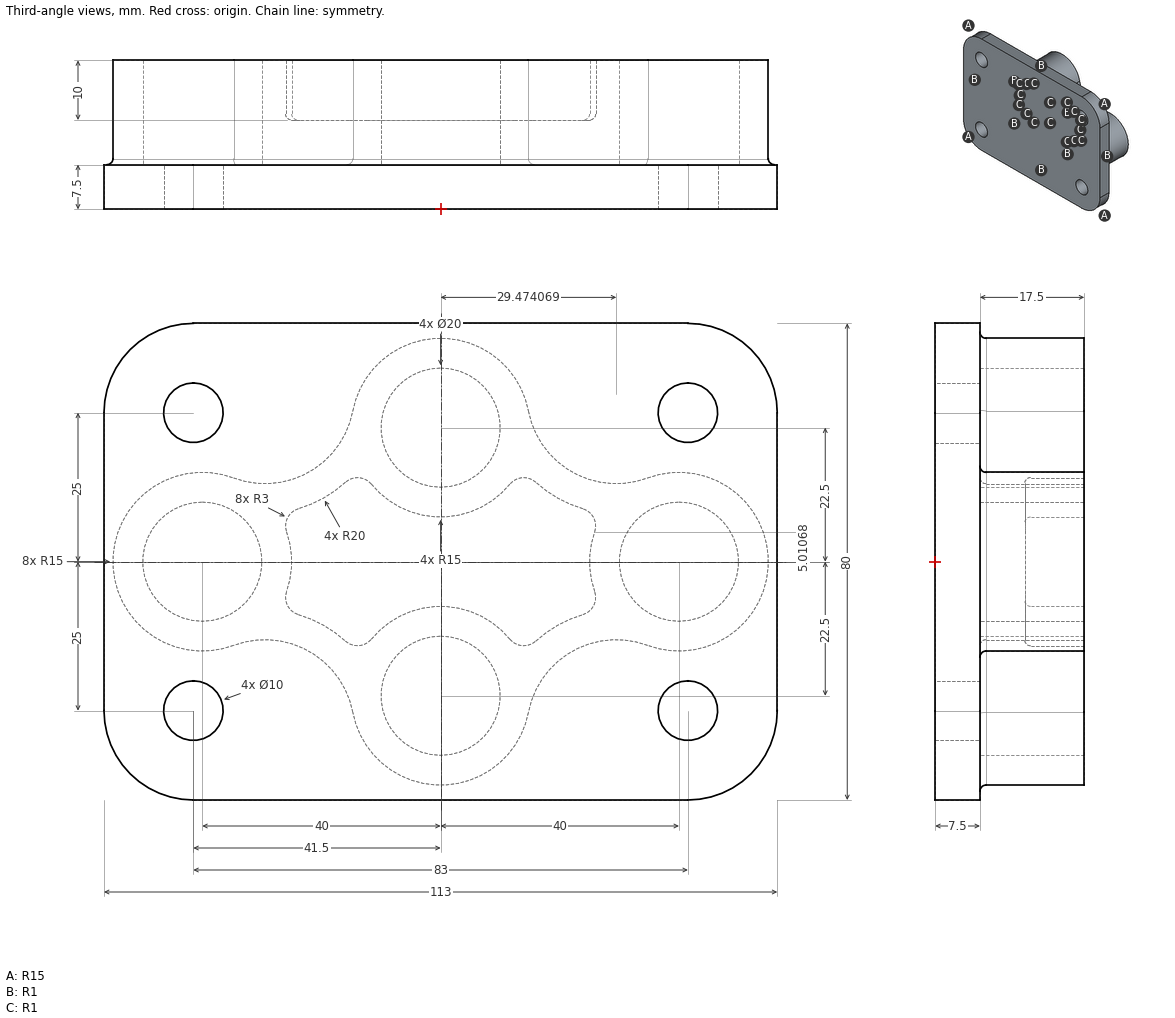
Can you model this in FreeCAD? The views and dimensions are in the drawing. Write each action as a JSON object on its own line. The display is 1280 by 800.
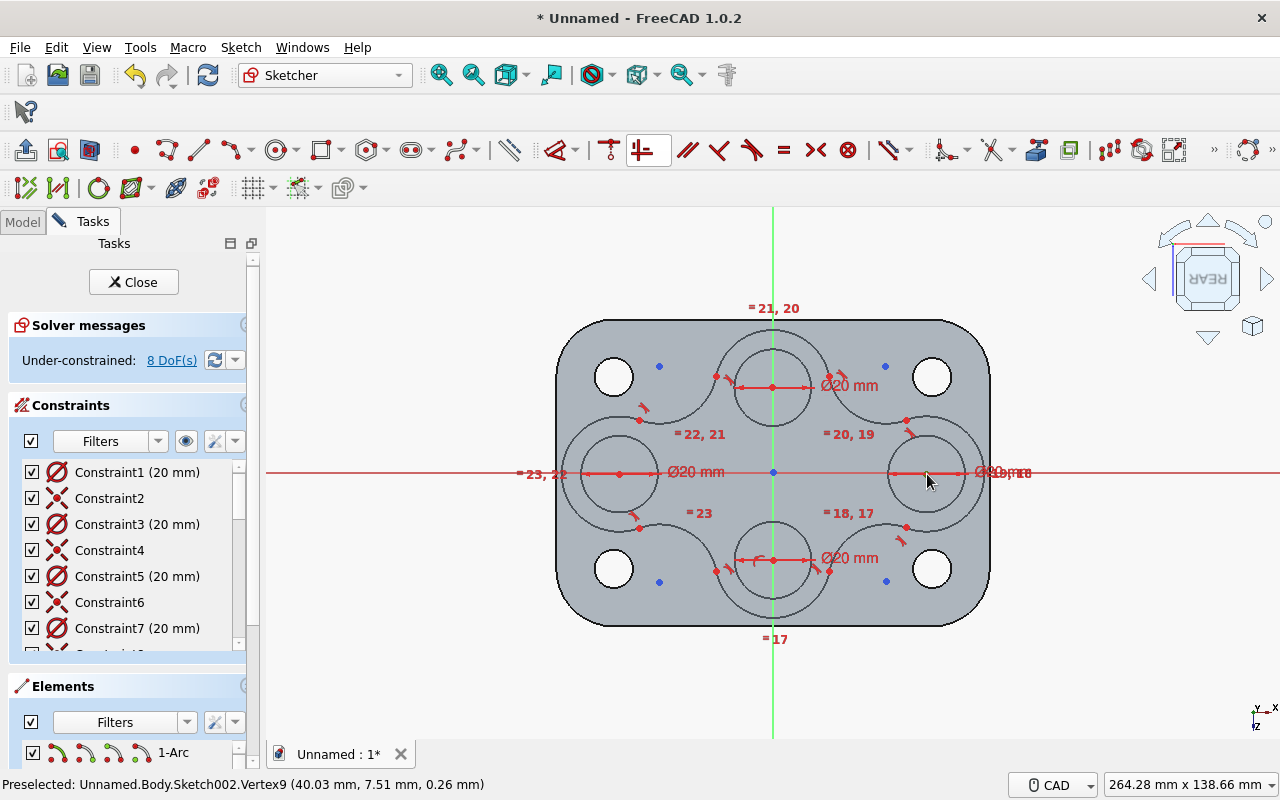
{"action": "left_click", "coordinate": [353, 473]}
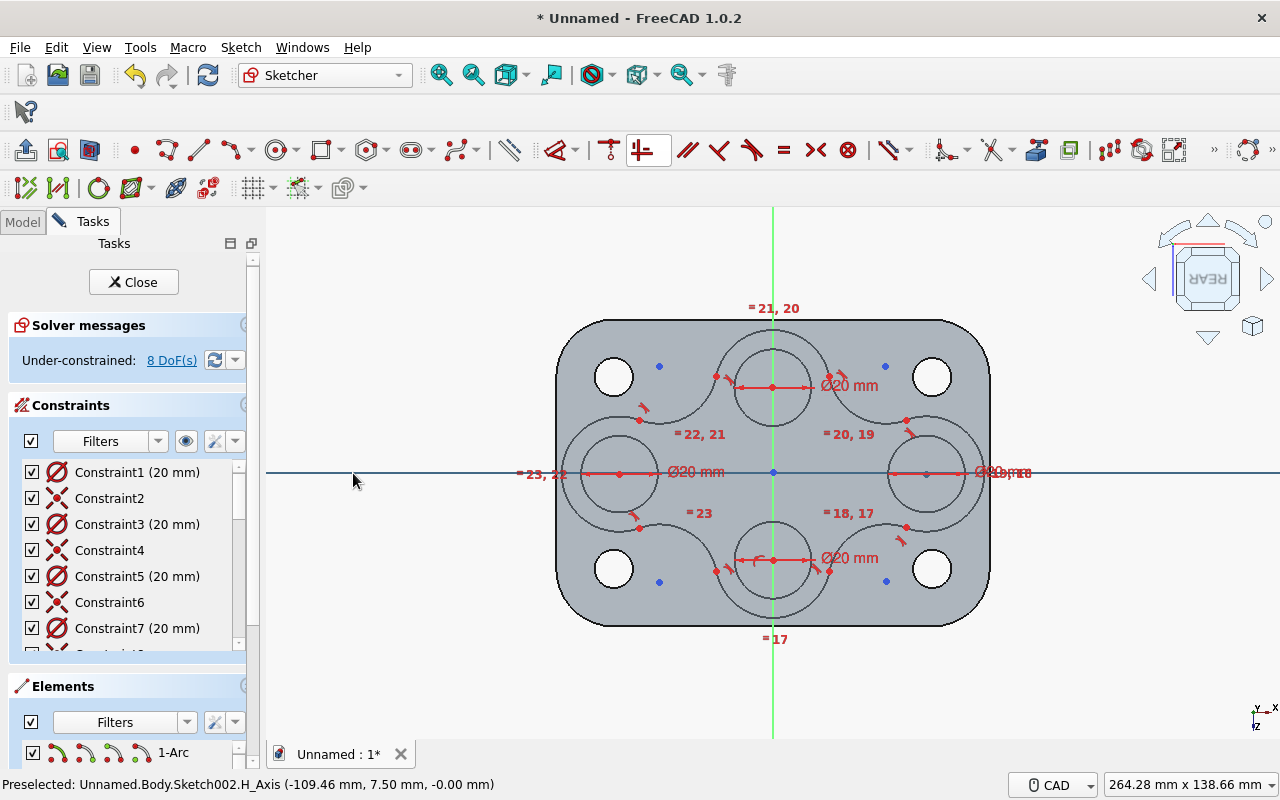
{"action": "left_click", "coordinate": [610, 150]}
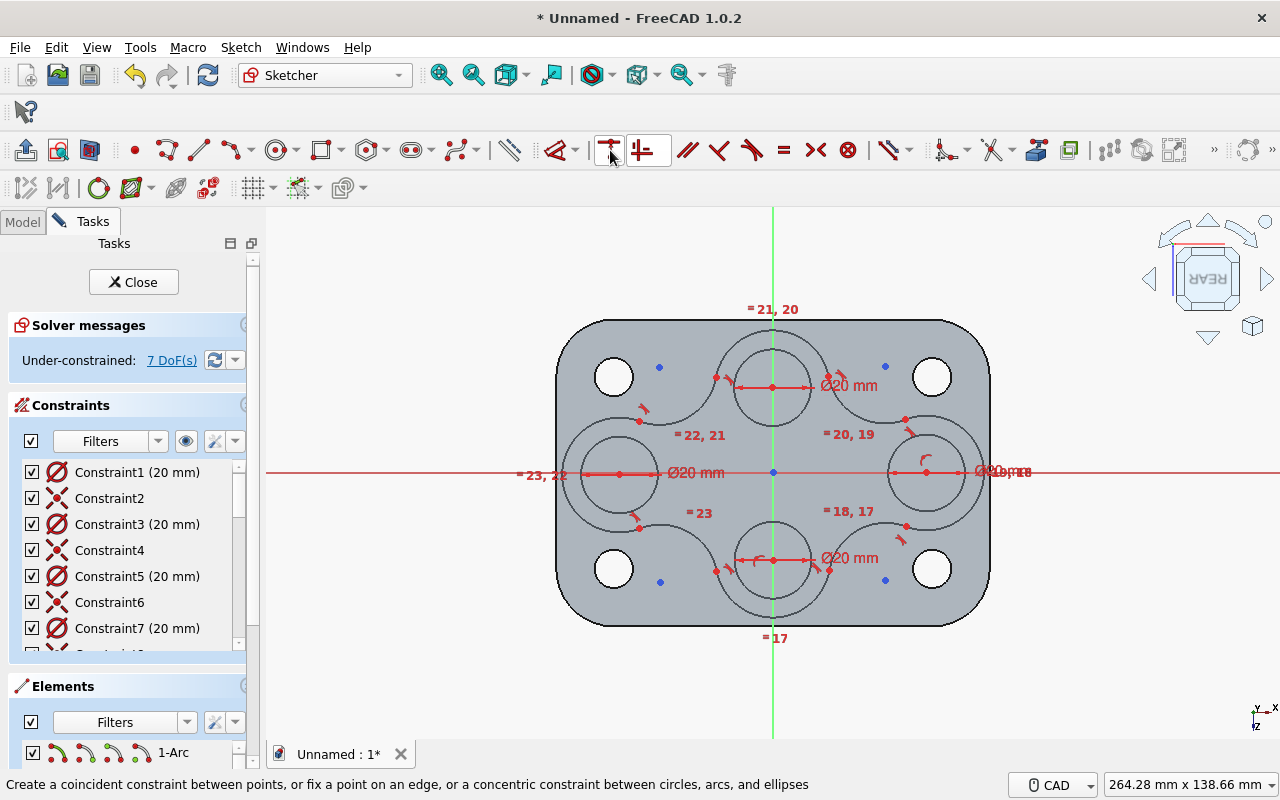
{"action": "left_click", "coordinate": [772, 388]}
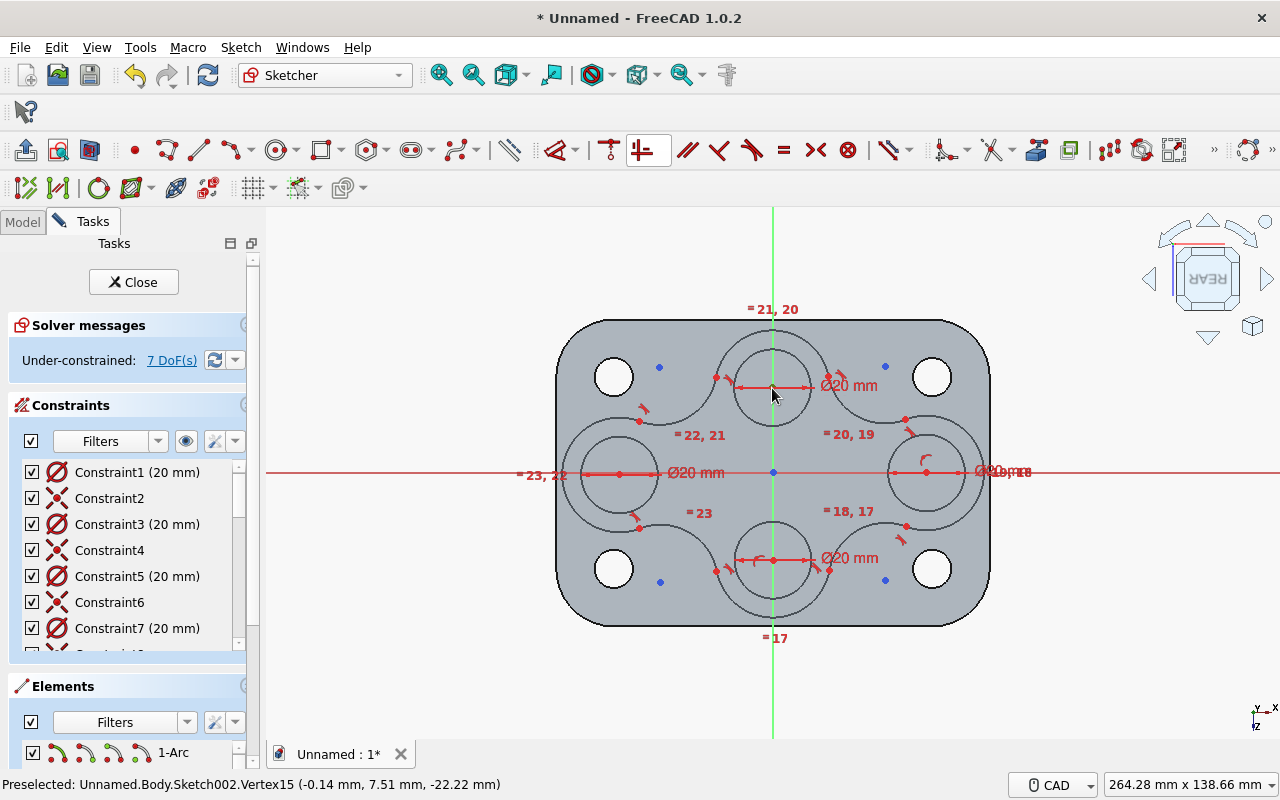
{"action": "left_click", "coordinate": [773, 677]}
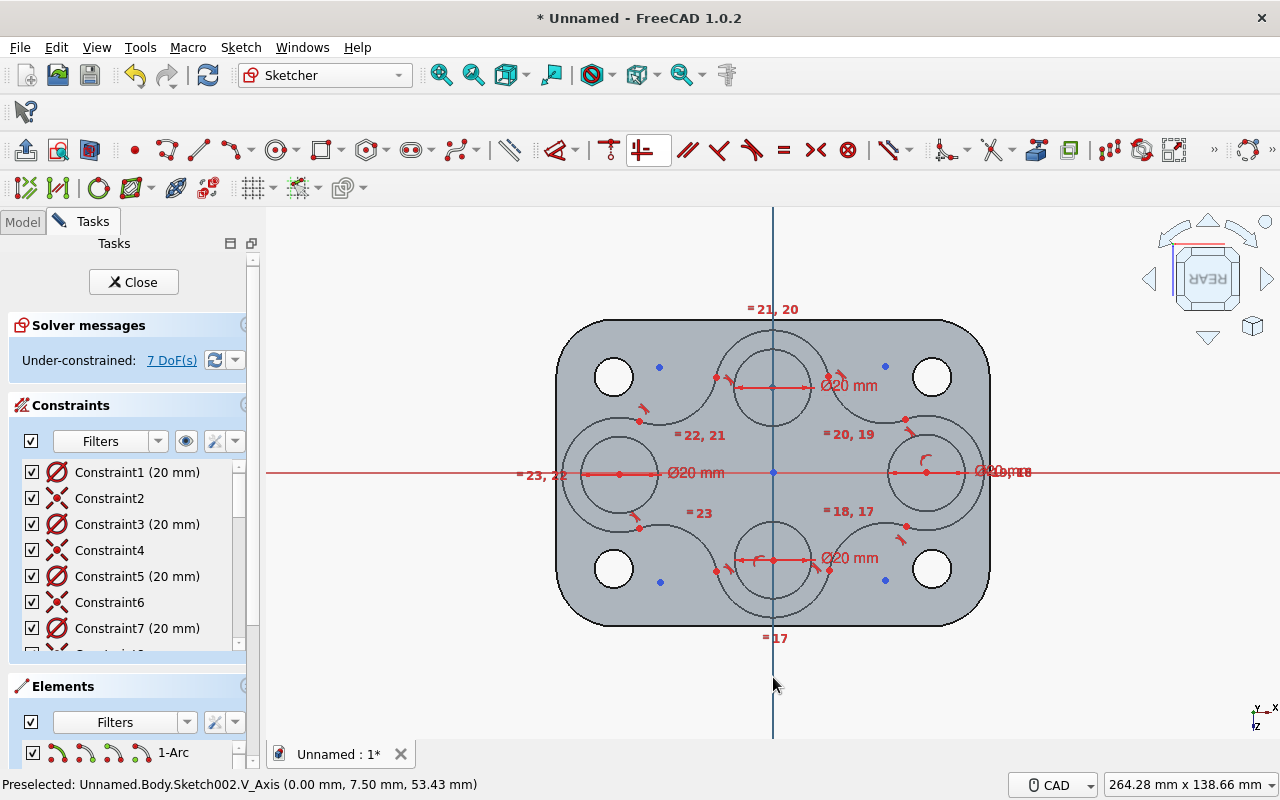
{"action": "left_click", "coordinate": [610, 150]}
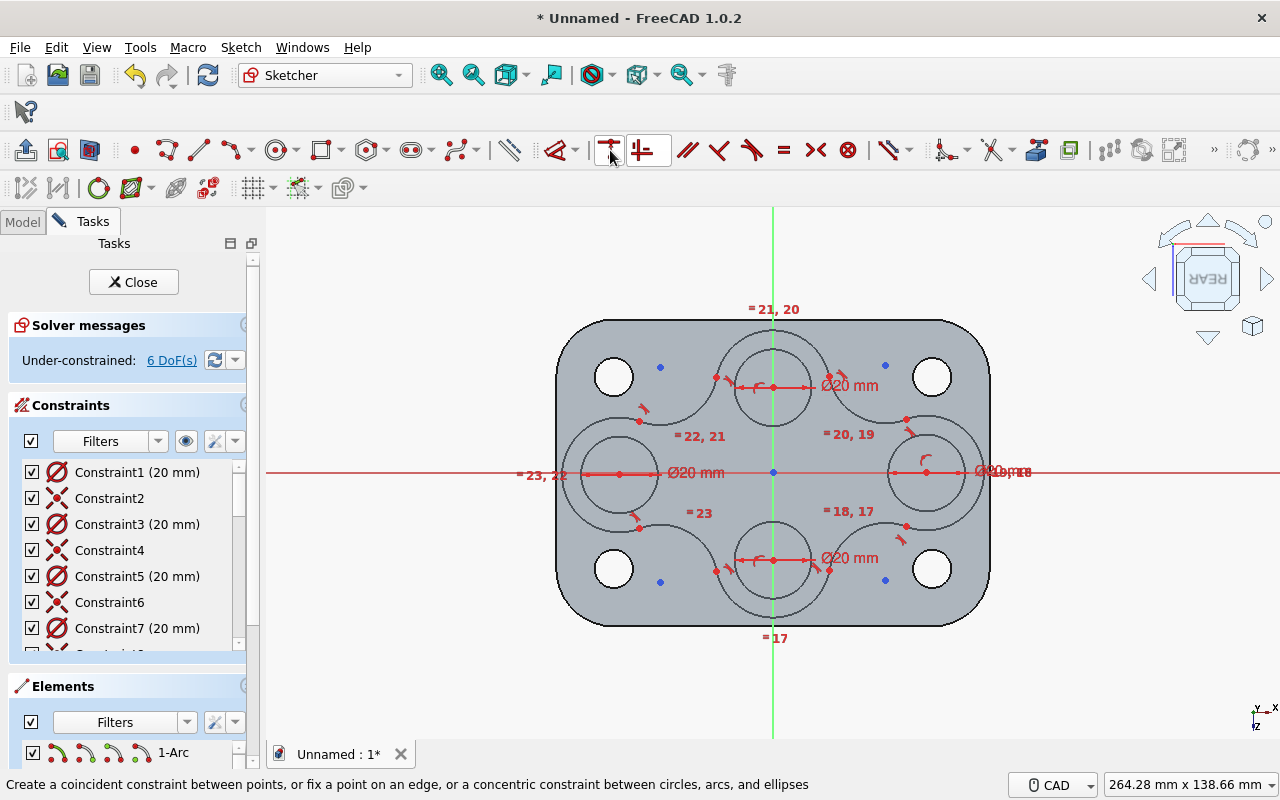
{"action": "left_click", "coordinate": [619, 475]}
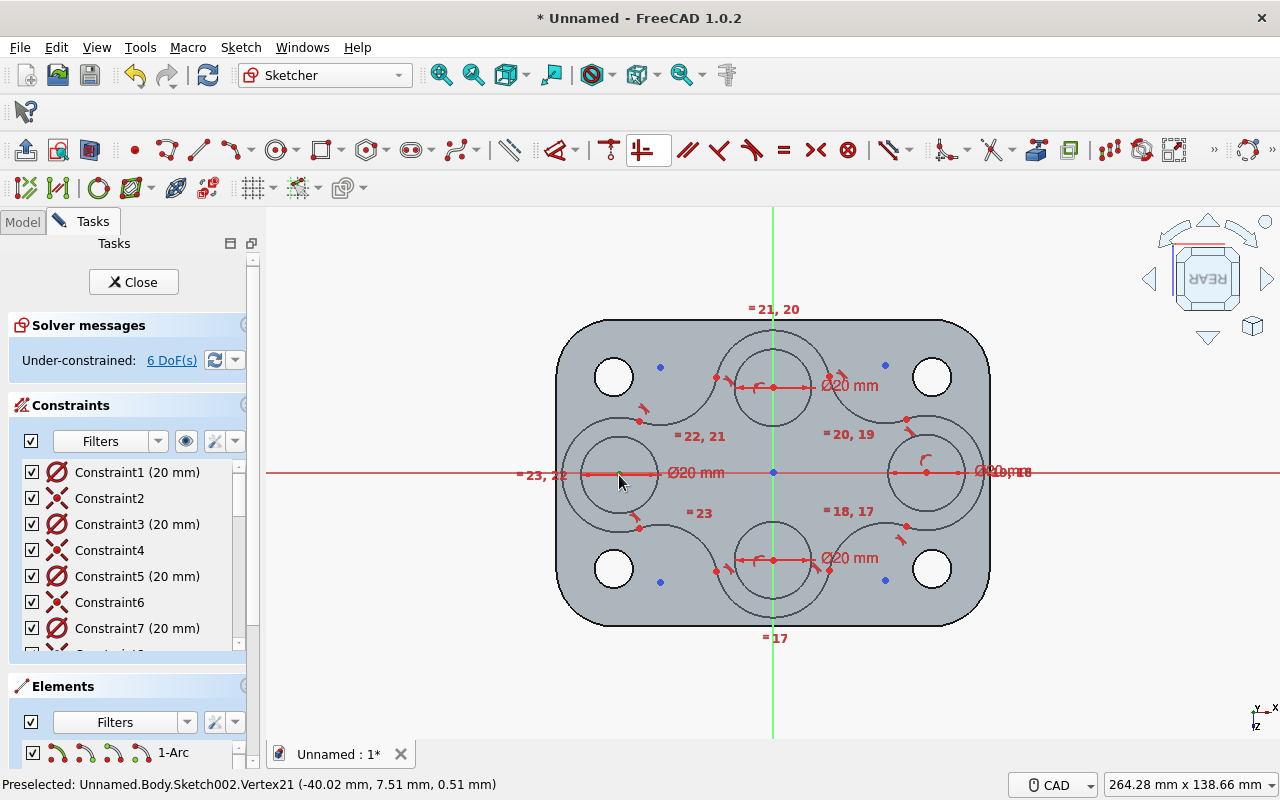
{"action": "left_click", "coordinate": [353, 473]}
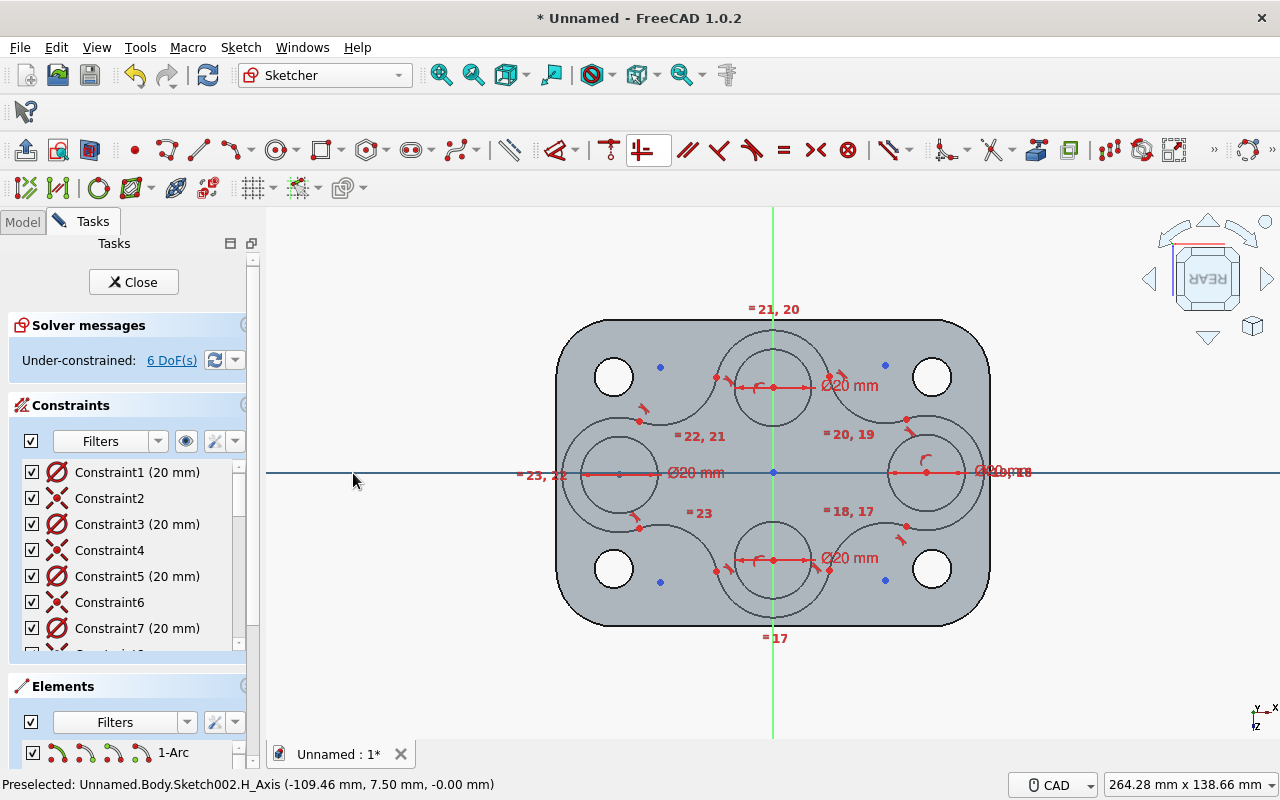
{"action": "key", "text": "c"}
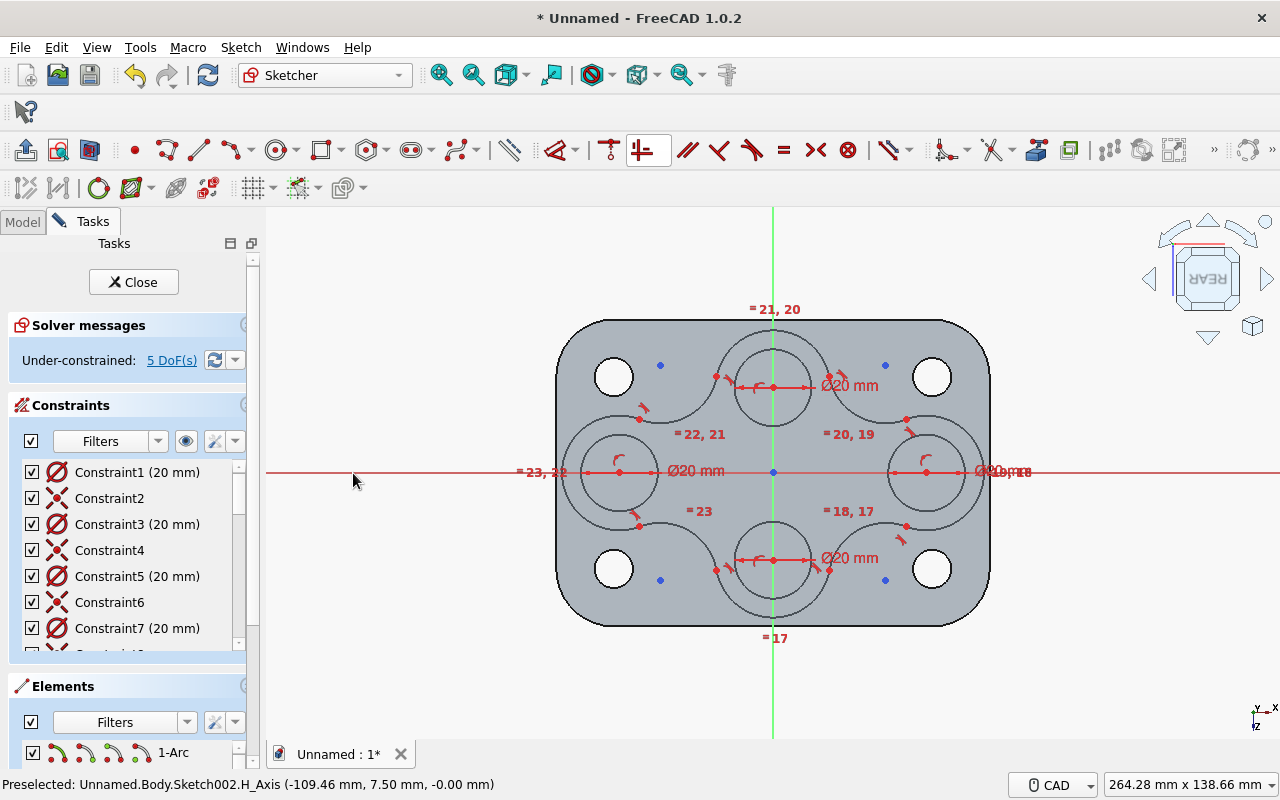
{"action": "left_click", "coordinate": [556, 150]}